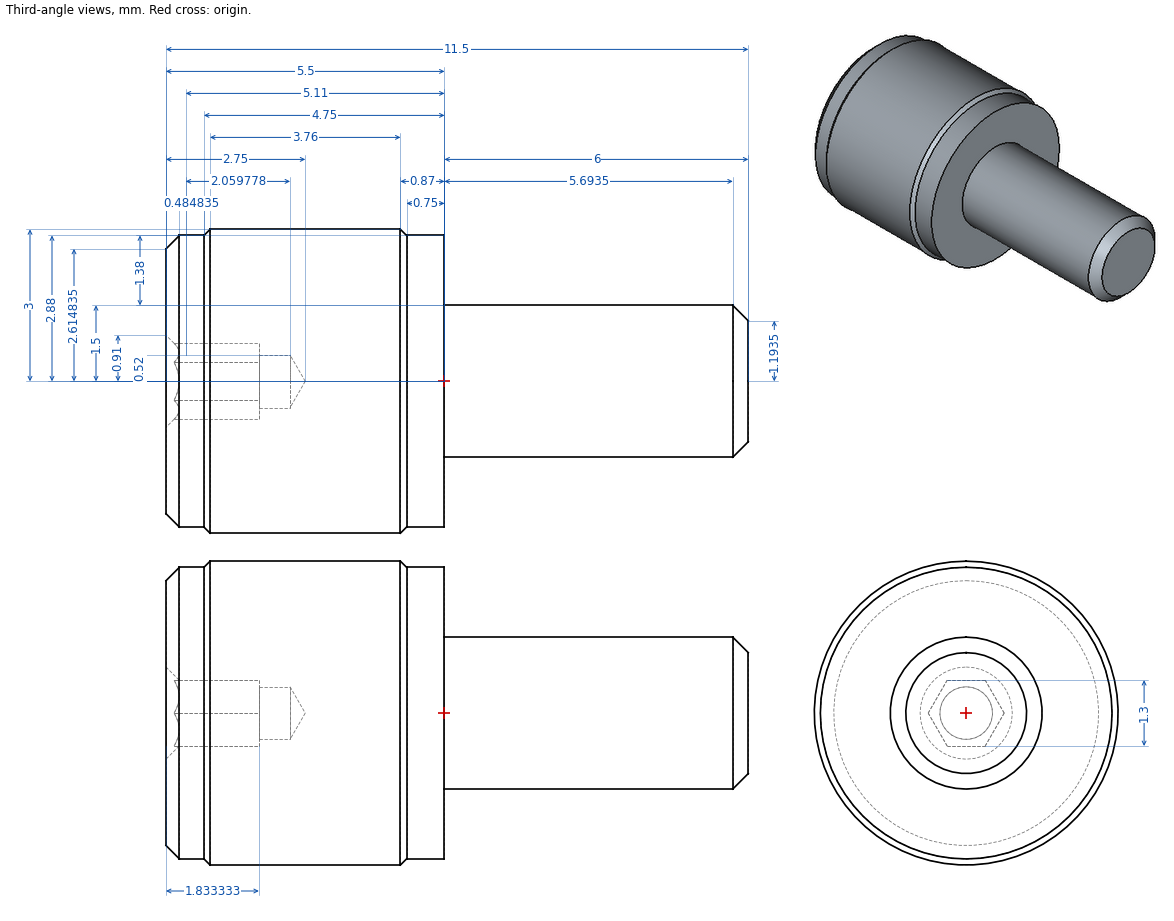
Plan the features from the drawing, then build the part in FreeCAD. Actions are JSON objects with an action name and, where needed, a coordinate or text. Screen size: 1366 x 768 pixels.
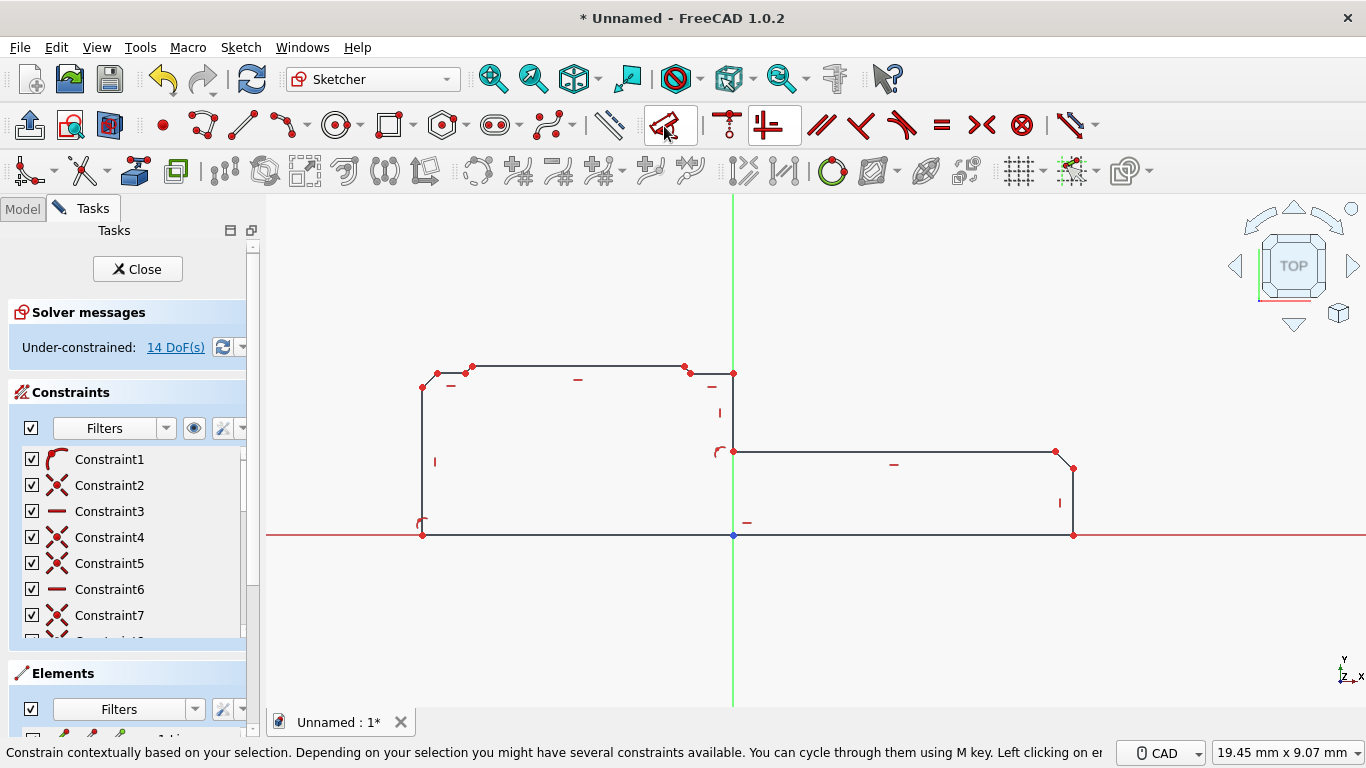
{"action": "scroll", "coordinate": [684, 366], "scroll_direction": "up", "scroll_amount": 2}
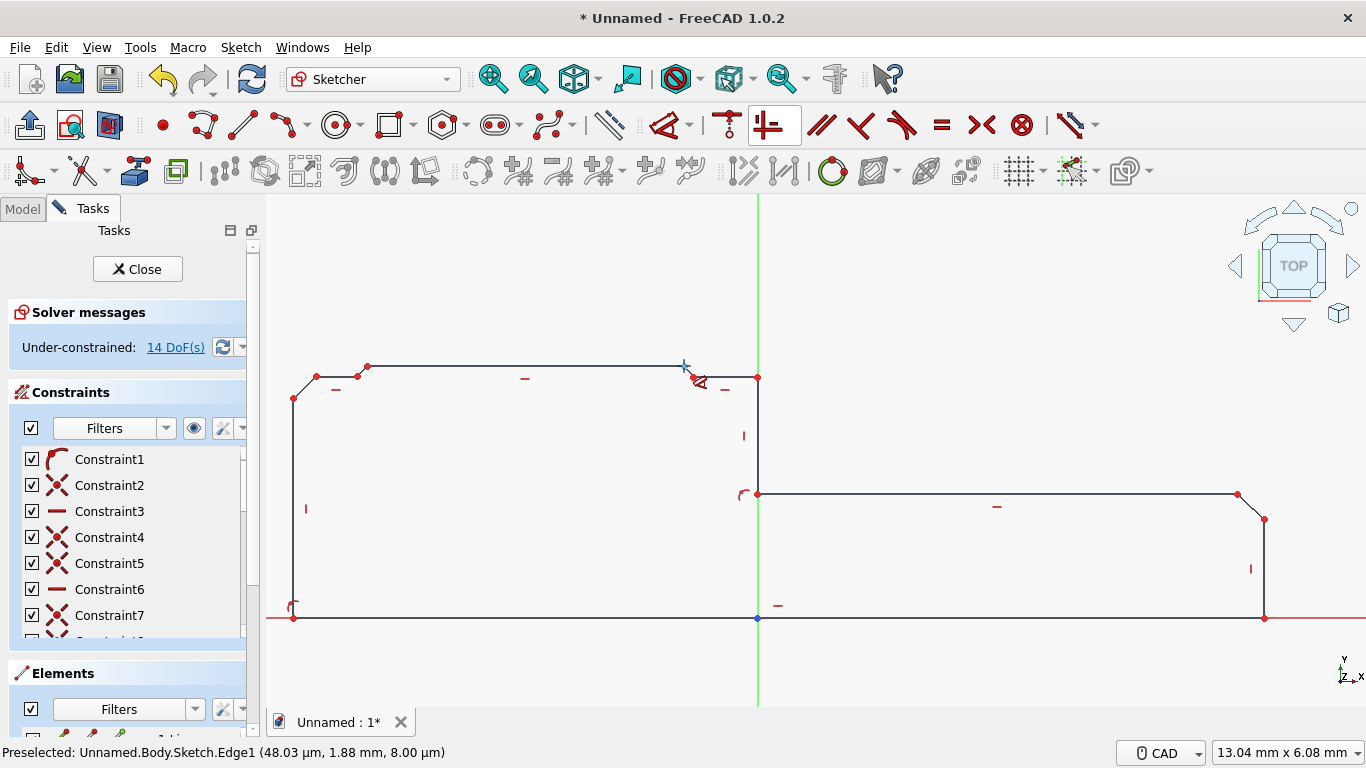
{"action": "left_click", "coordinate": [684, 366]}
{"action": "left_click", "coordinate": [650, 492]}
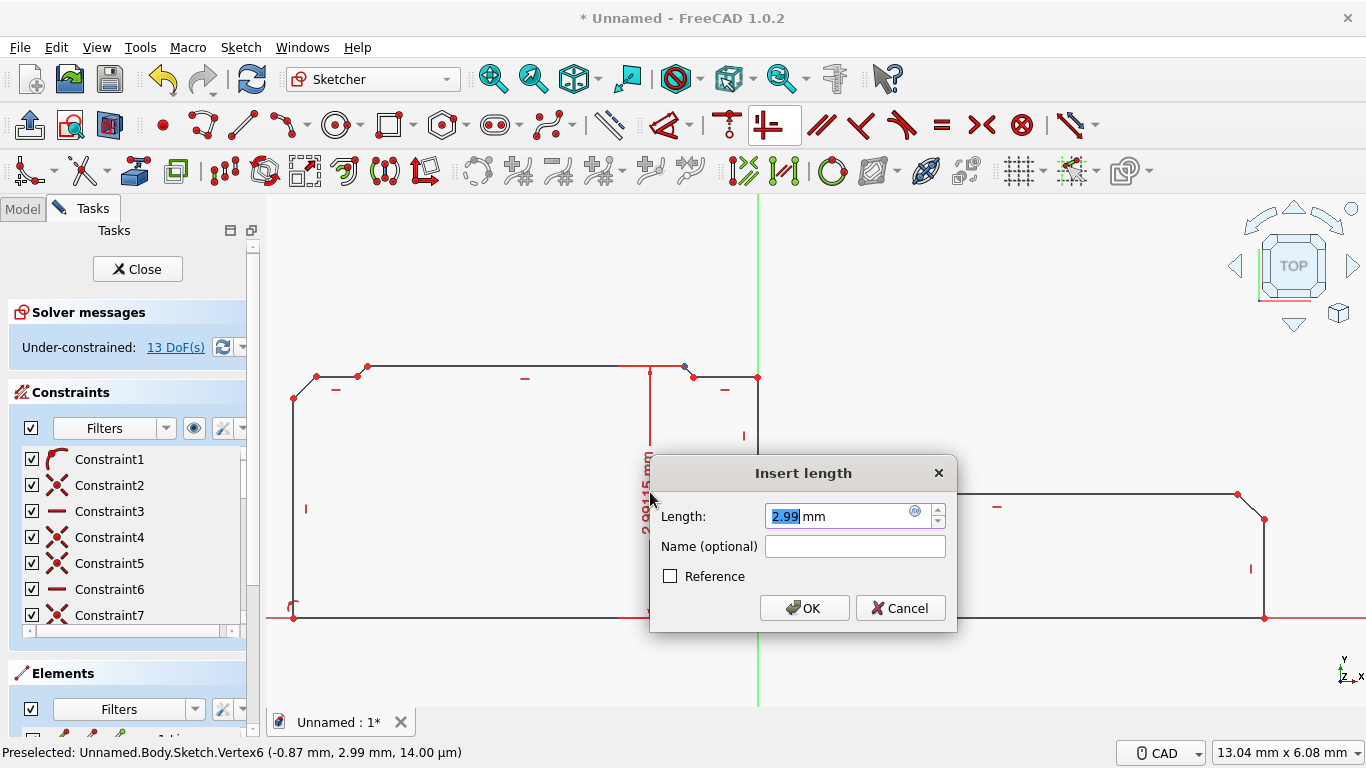
{"action": "type", "text": "3"}
{"action": "key", "text": "Return"}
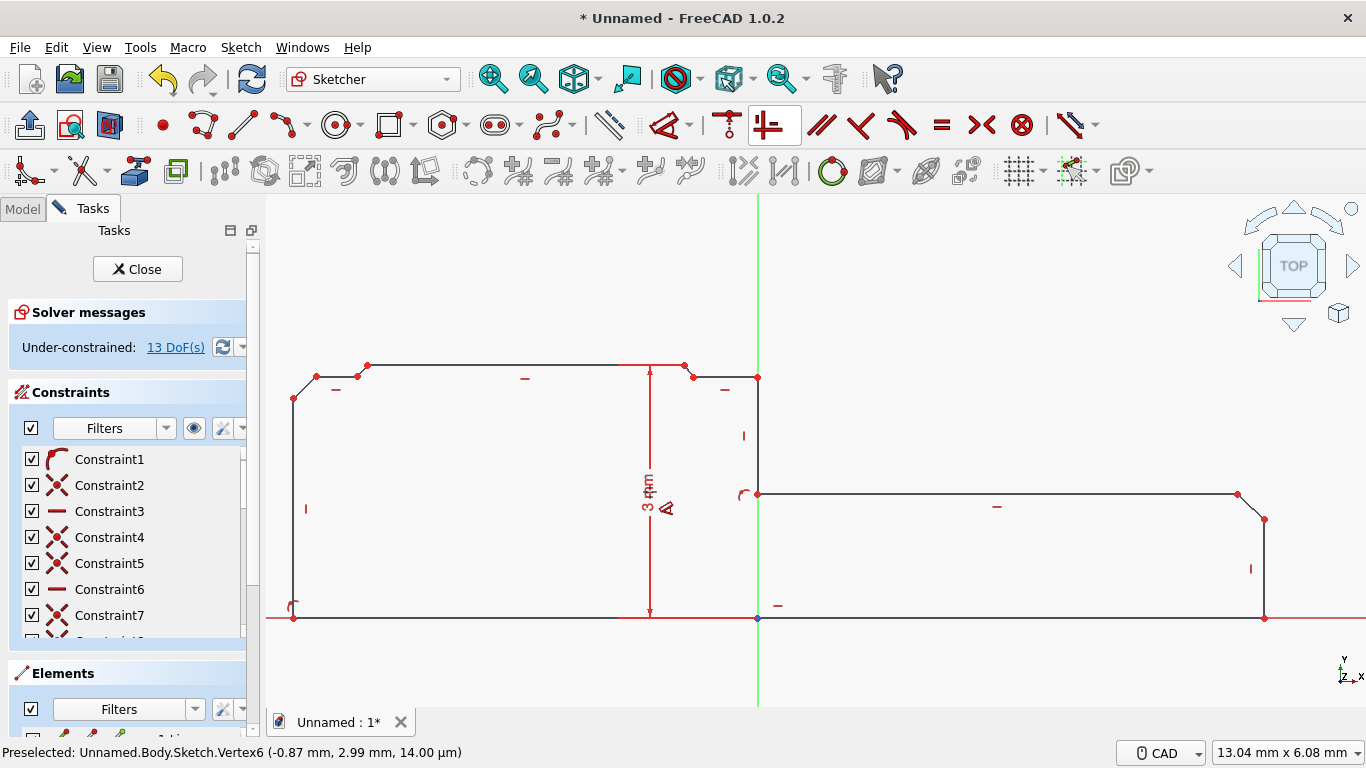
{"action": "scroll", "coordinate": [684, 366], "scroll_direction": "down", "scroll_amount": 2}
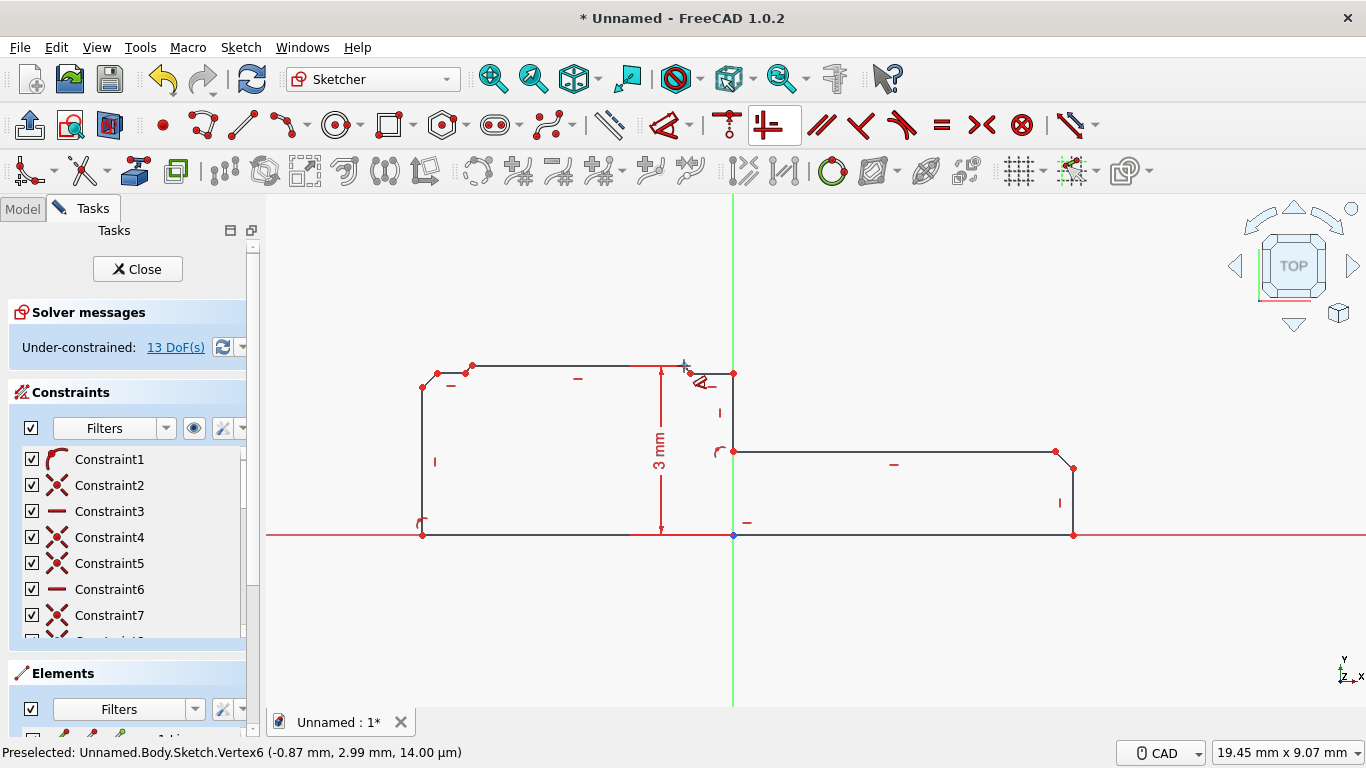
{"action": "left_click", "coordinate": [1073, 535]}
{"action": "left_click", "coordinate": [903, 569]}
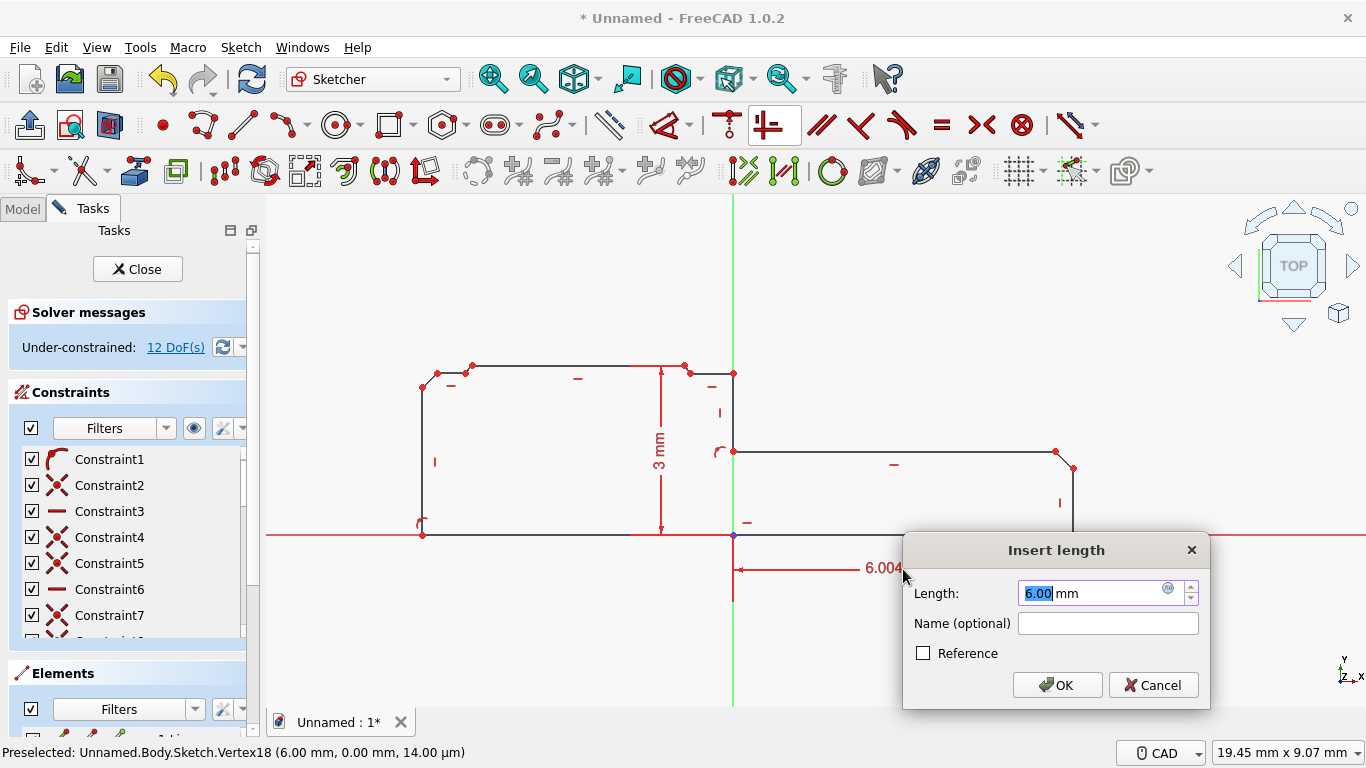
{"action": "type", "text": "6"}
{"action": "key", "text": "Return"}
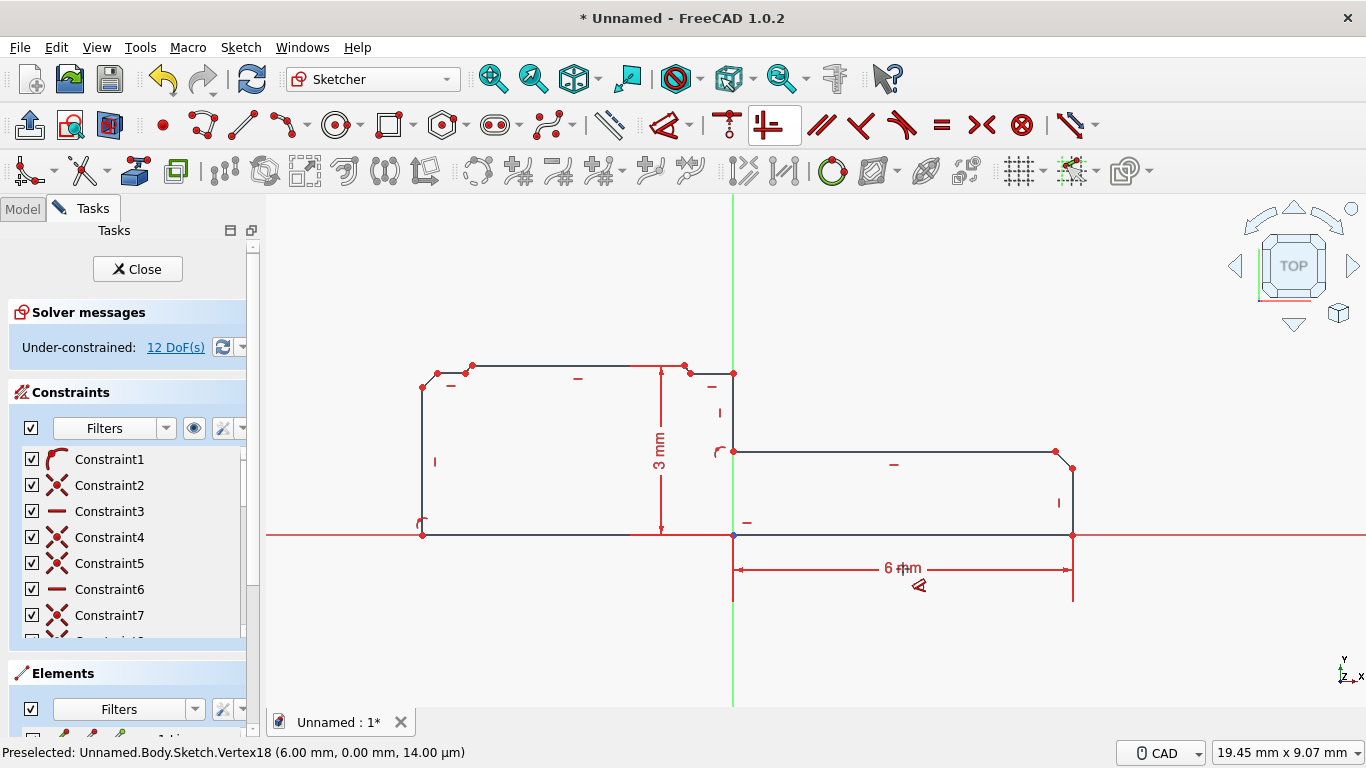
{"action": "left_click", "coordinate": [733, 428]}
{"action": "left_click", "coordinate": [699, 413]}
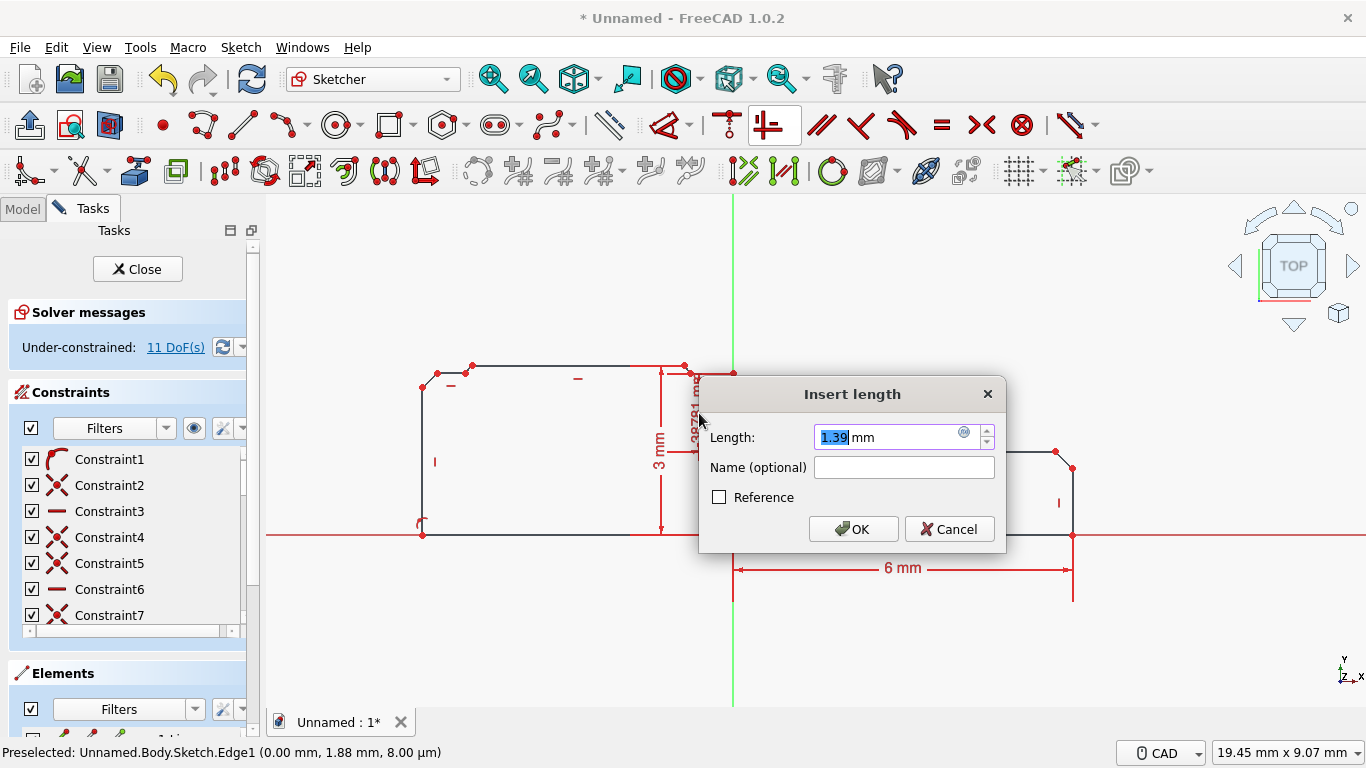
{"action": "type", "text": "1.38"}
{"action": "key", "text": "Return"}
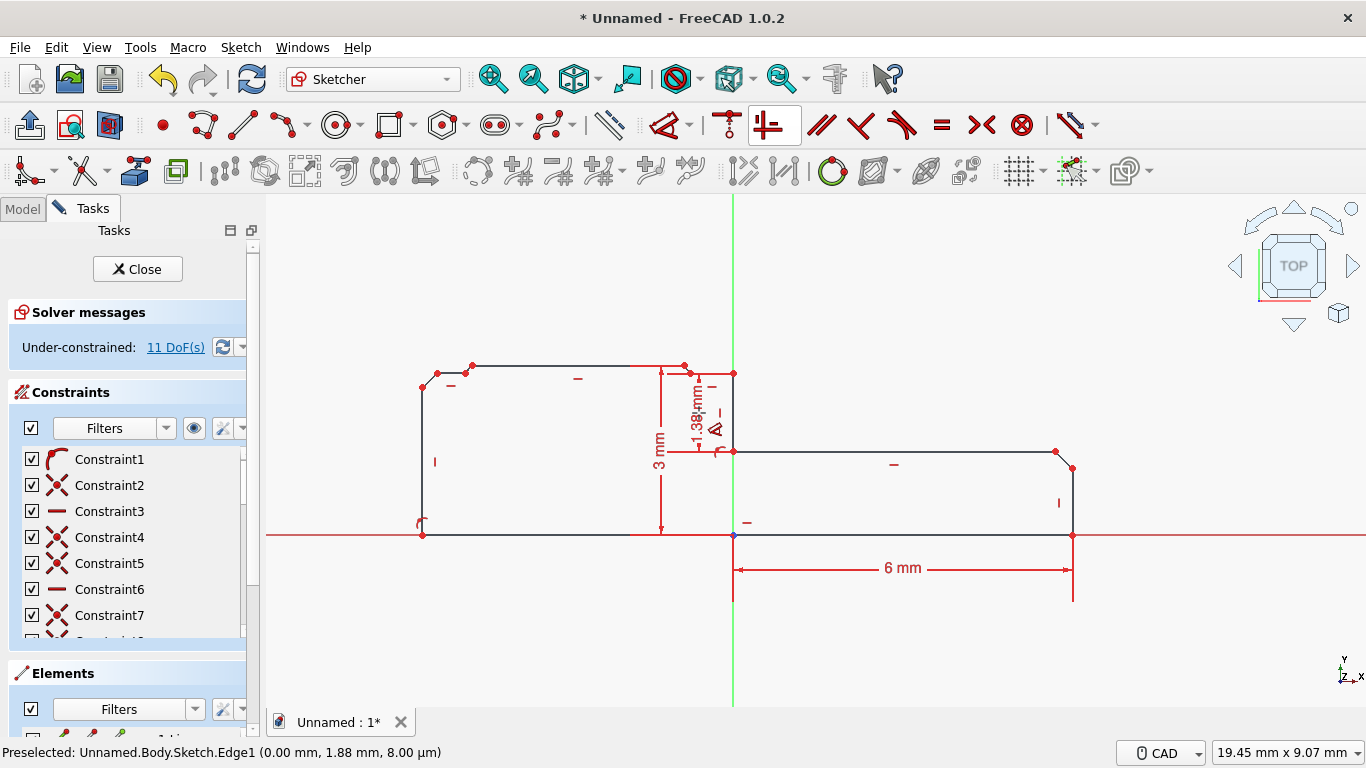
{"action": "left_click", "coordinate": [721, 374]}
{"action": "left_click", "coordinate": [712, 340]}